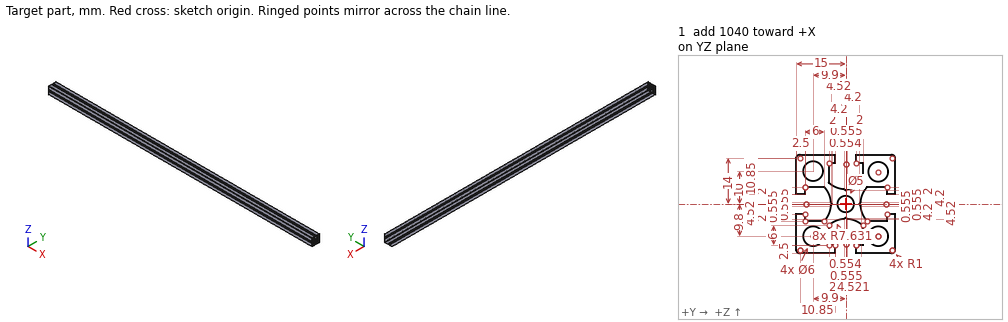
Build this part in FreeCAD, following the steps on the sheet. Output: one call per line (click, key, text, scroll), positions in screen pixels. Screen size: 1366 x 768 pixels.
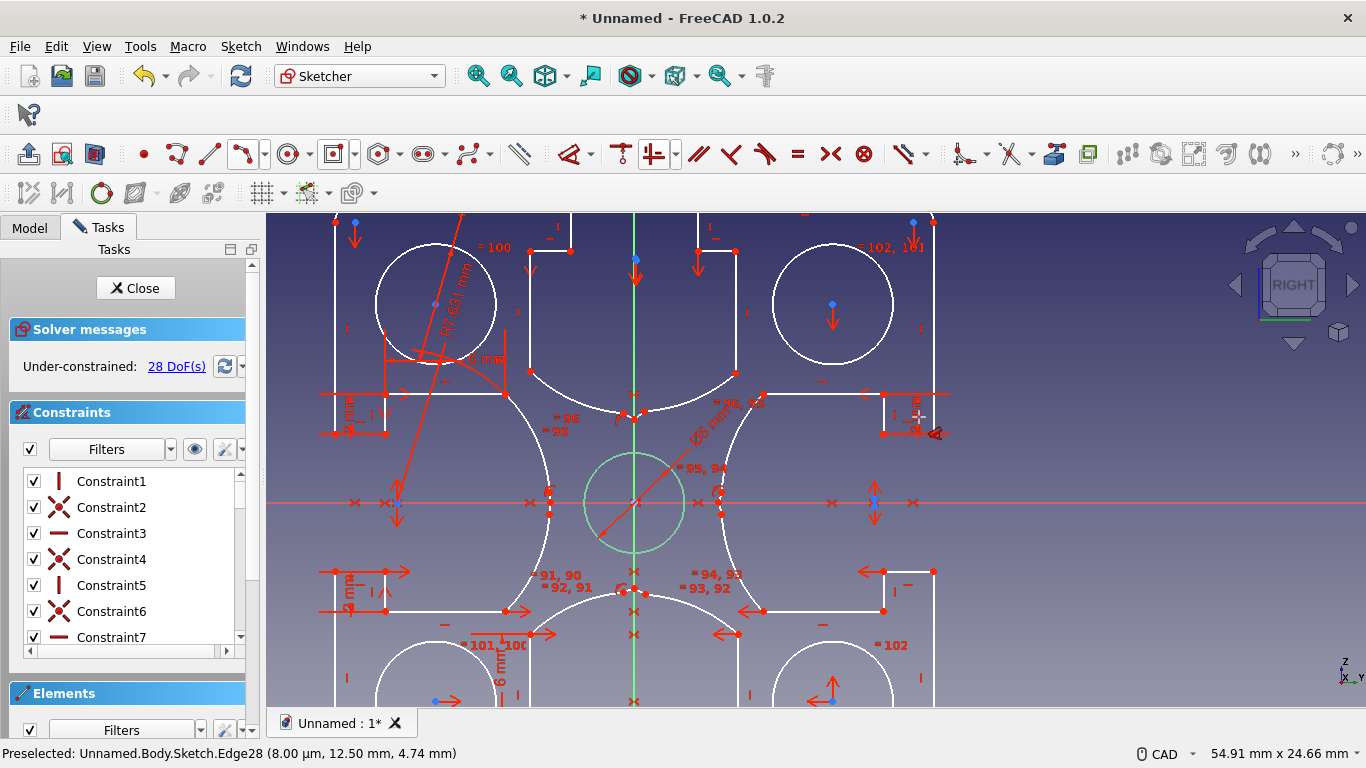
scroll(709, 251, up, 2)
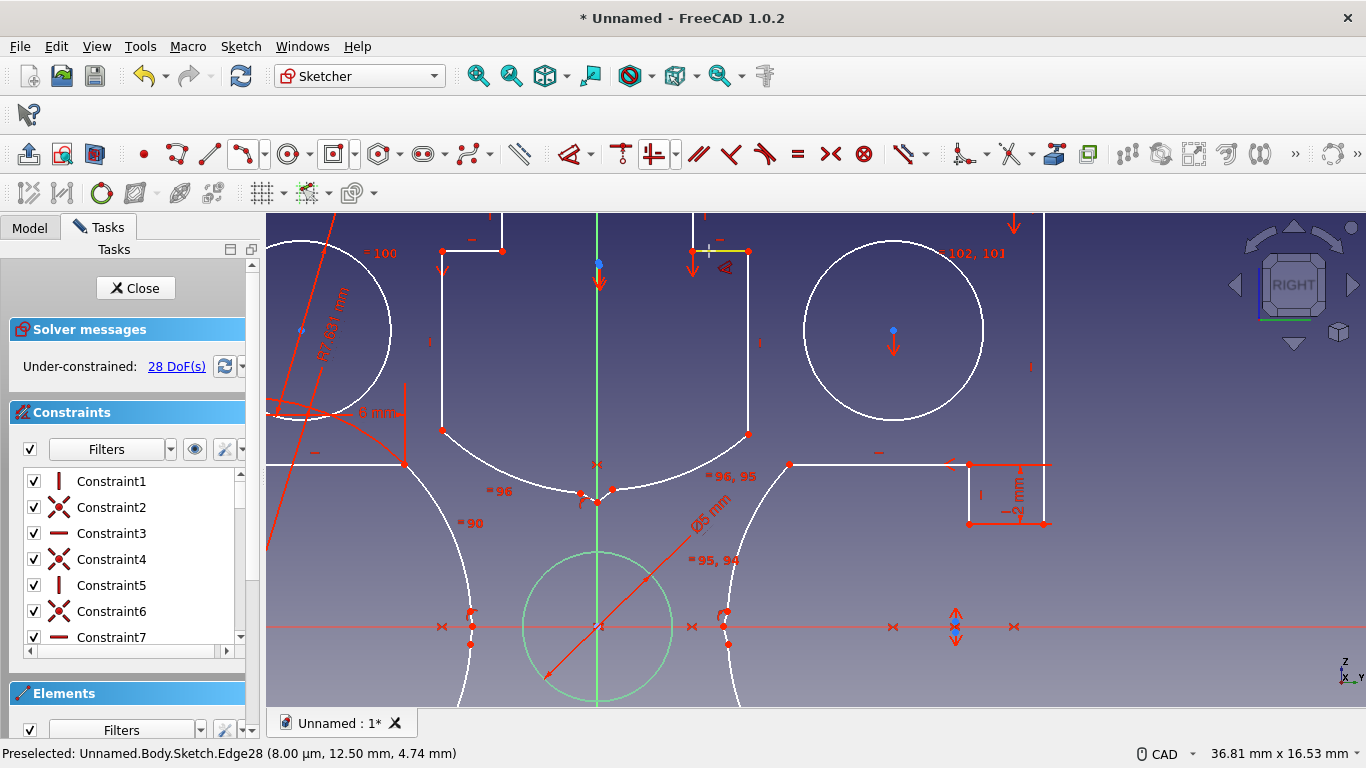
click(709, 251)
click(721, 285)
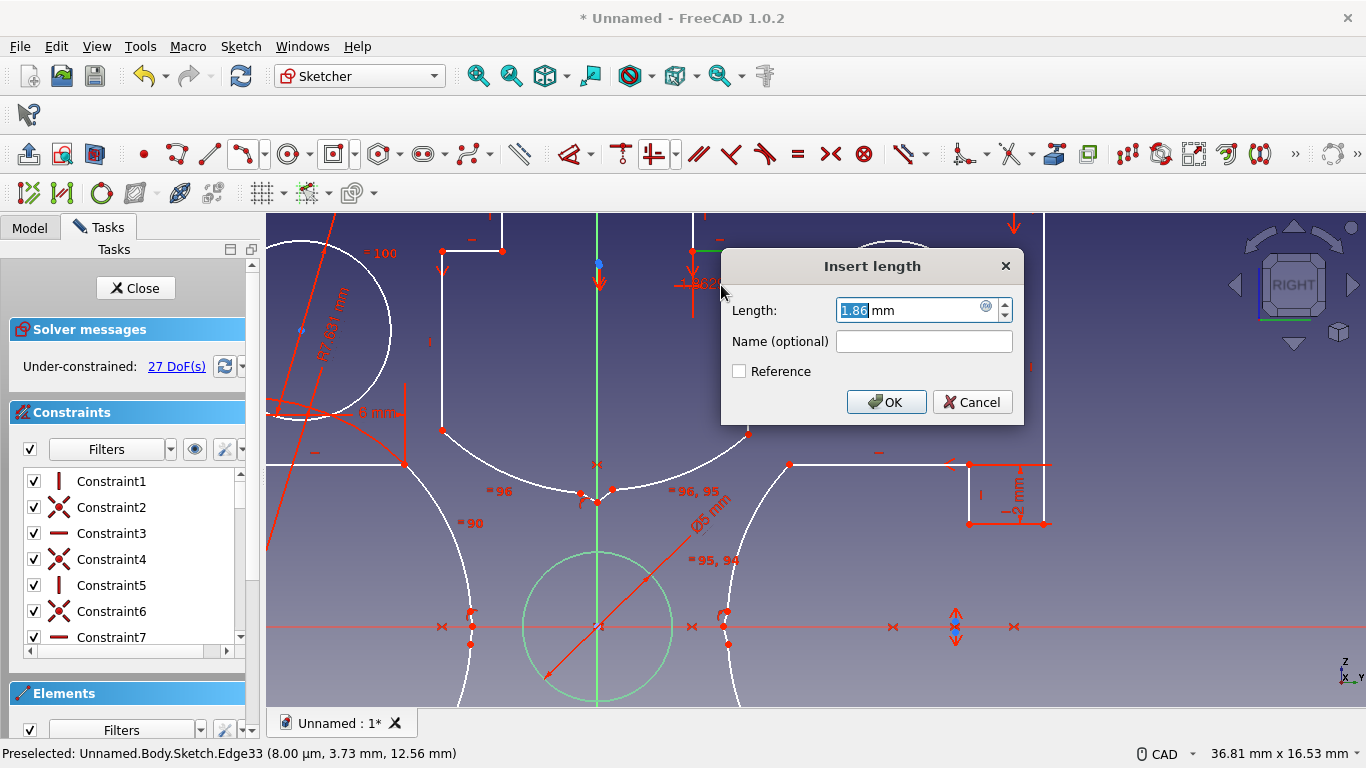
text(2)
key(Return)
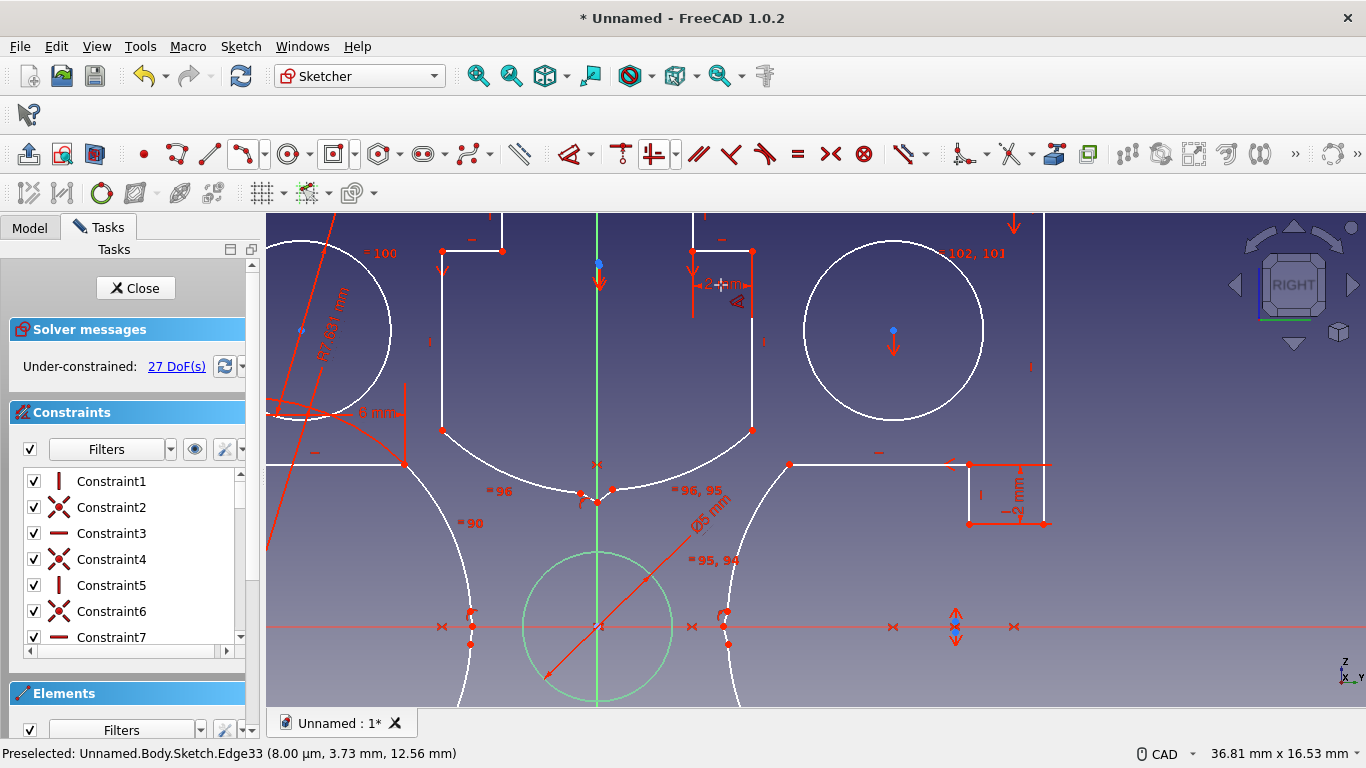
click(460, 251)
click(472, 285)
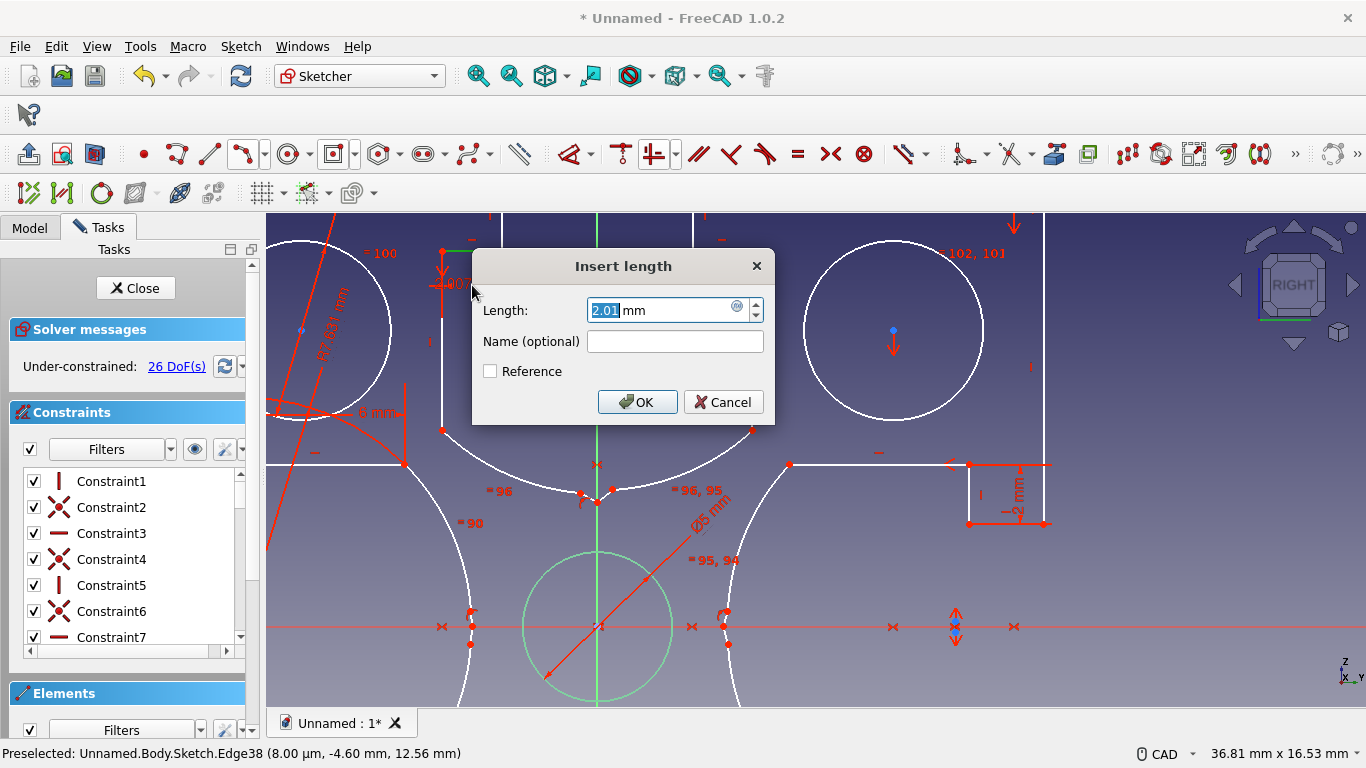
text(2)
key(Return)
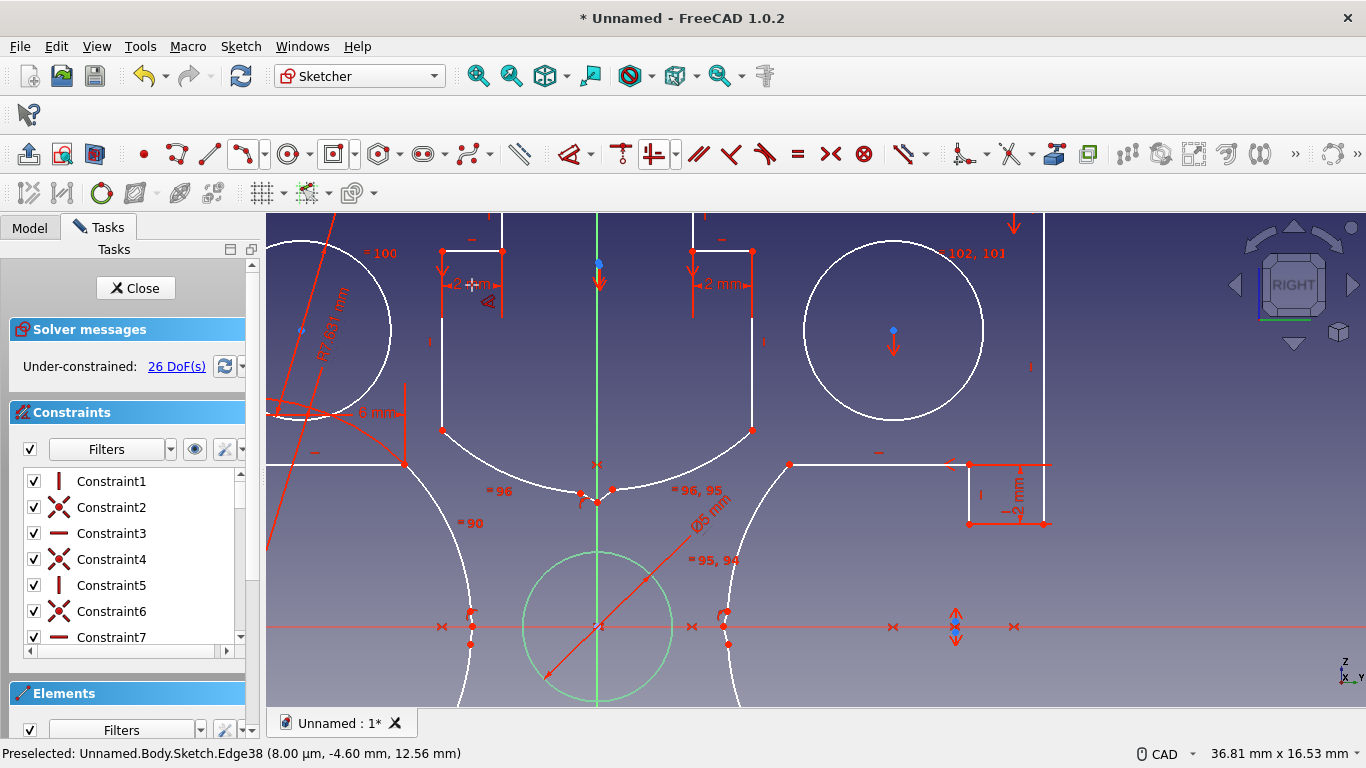
click(301, 331)
click(631, 411)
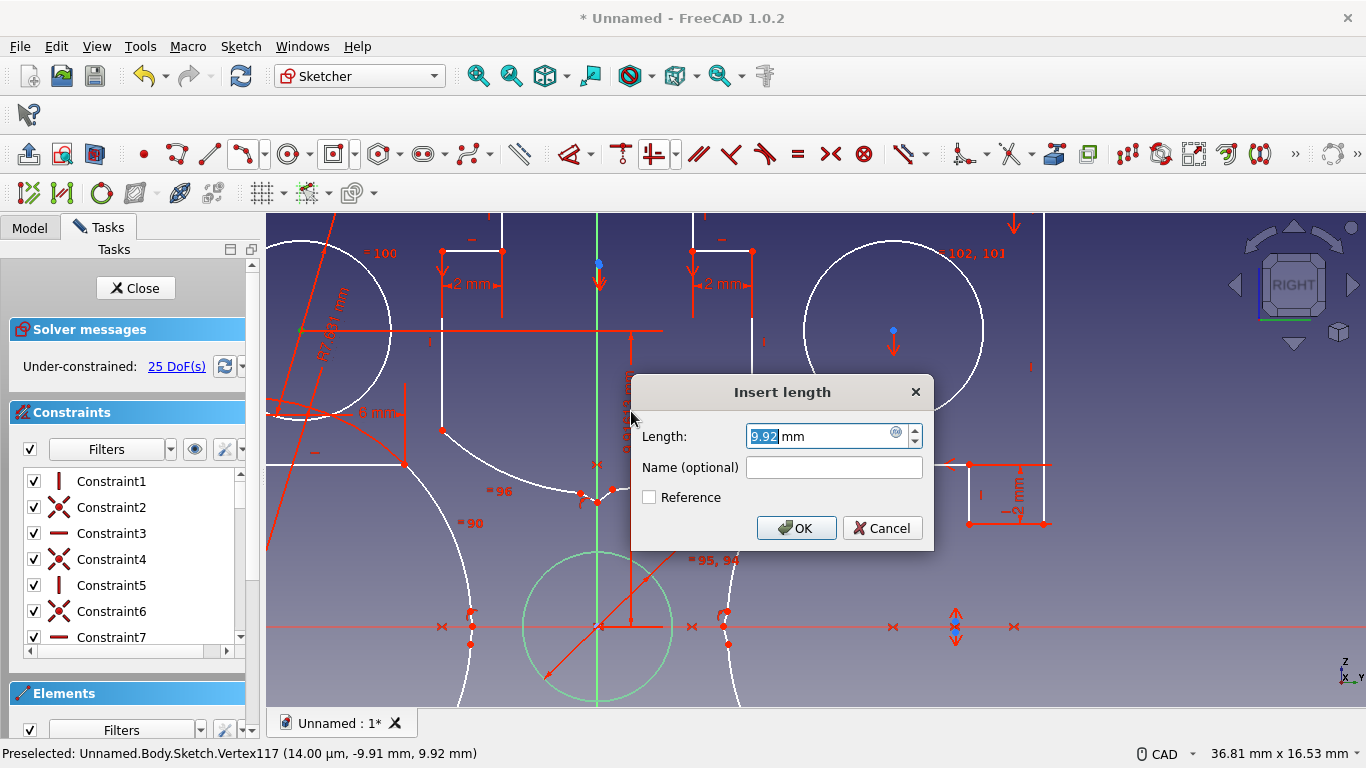
text(10)
key(Return)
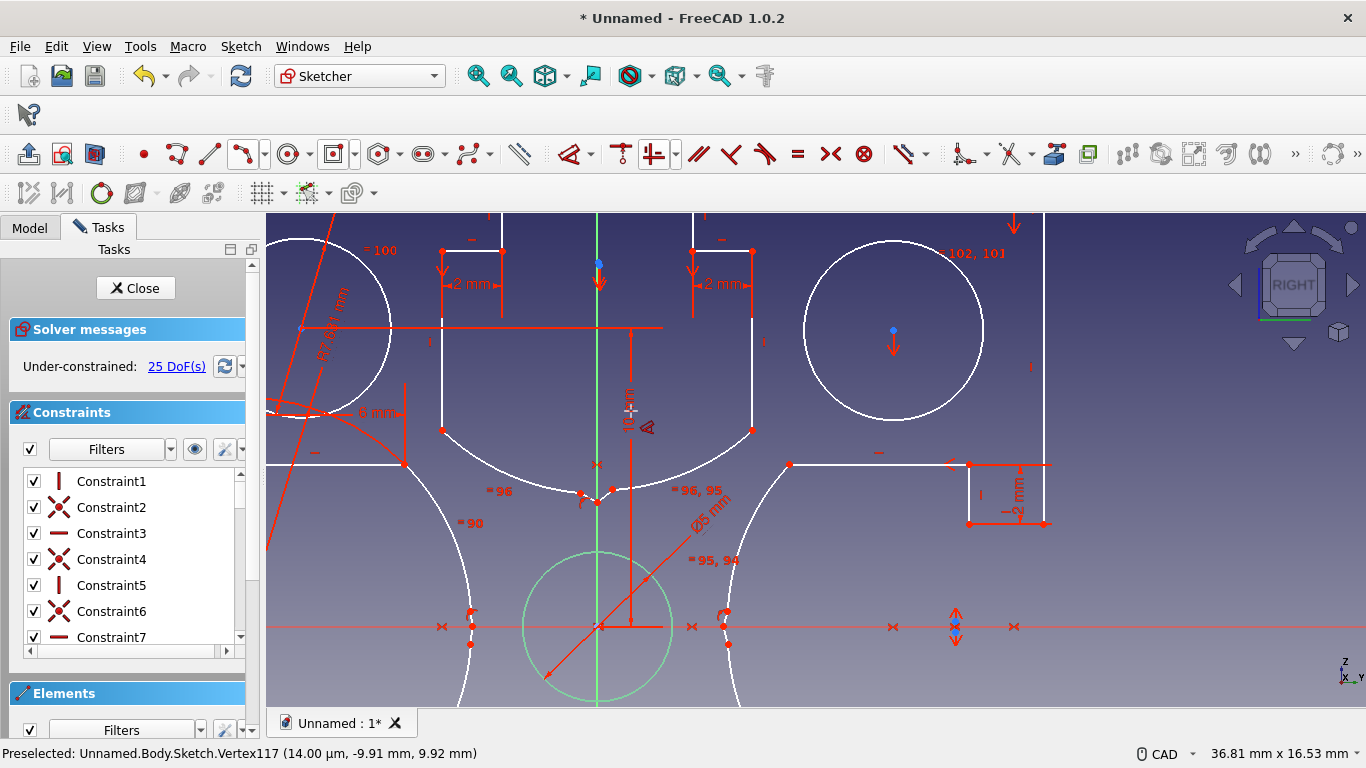
scroll(835, 363, down, 5)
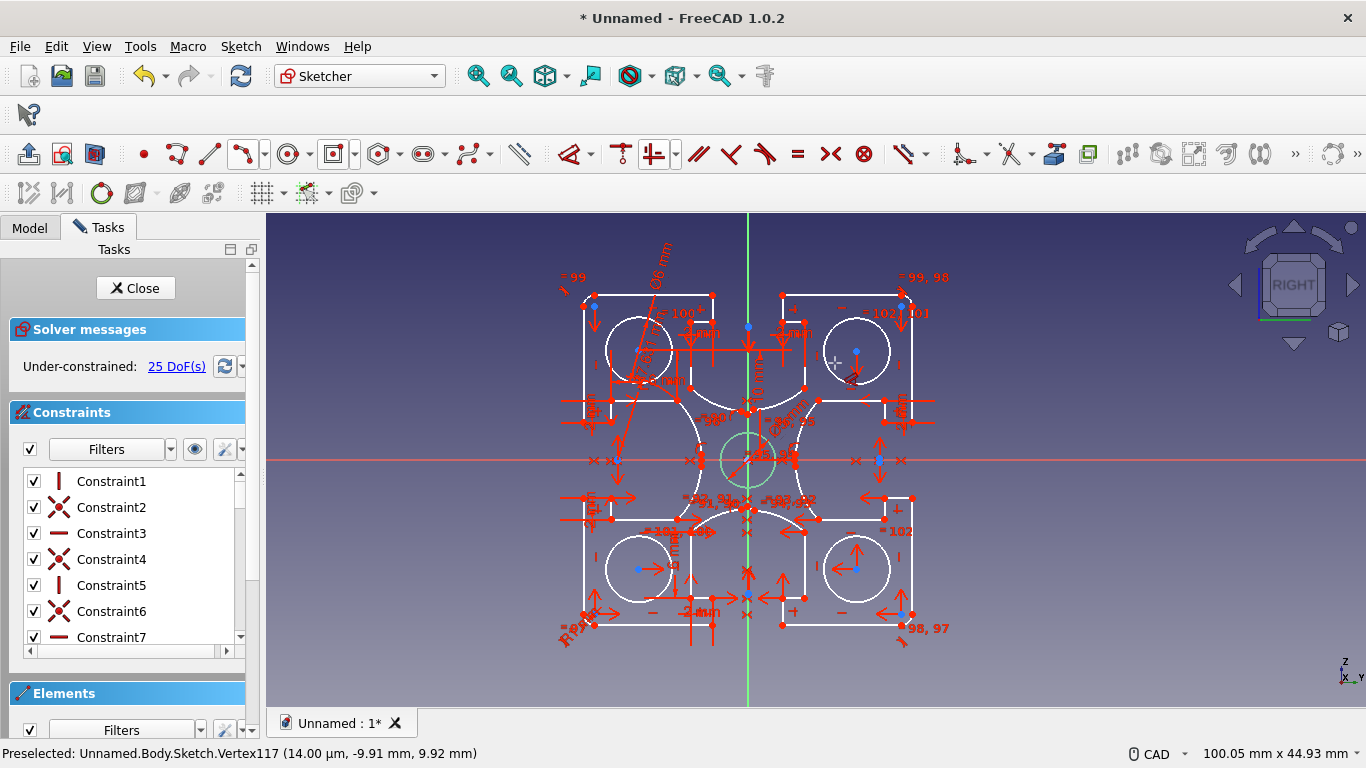
scroll(592, 423, up, 3)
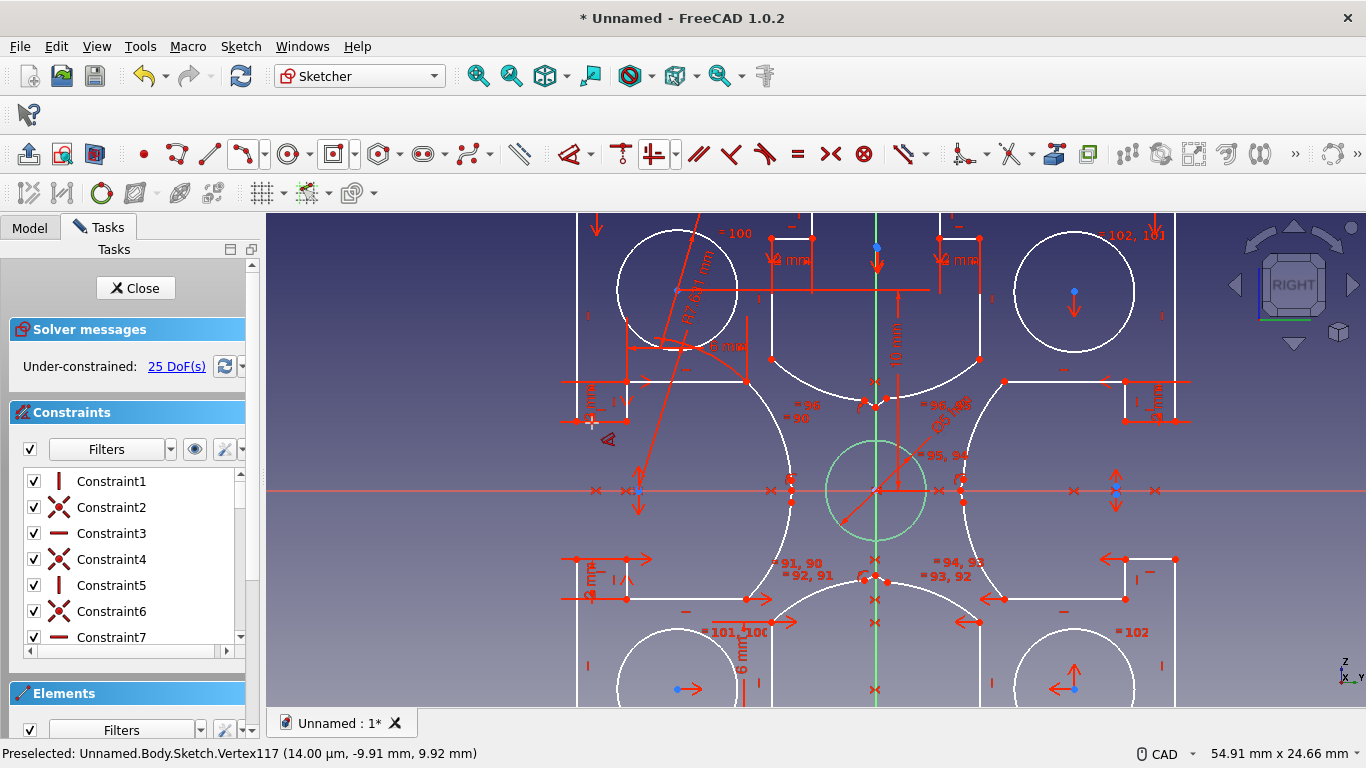
click(592, 422)
click(602, 456)